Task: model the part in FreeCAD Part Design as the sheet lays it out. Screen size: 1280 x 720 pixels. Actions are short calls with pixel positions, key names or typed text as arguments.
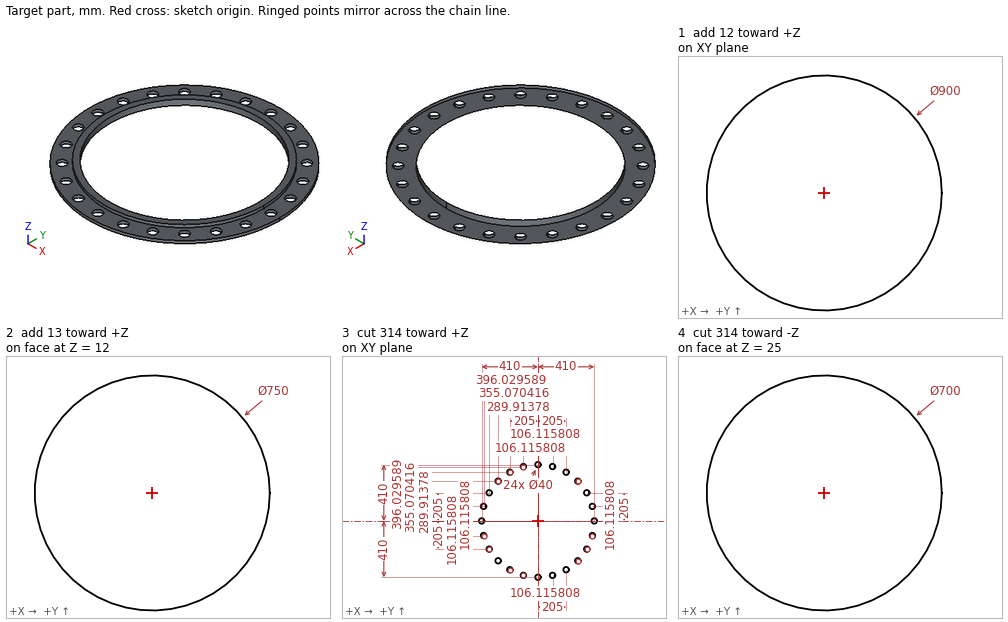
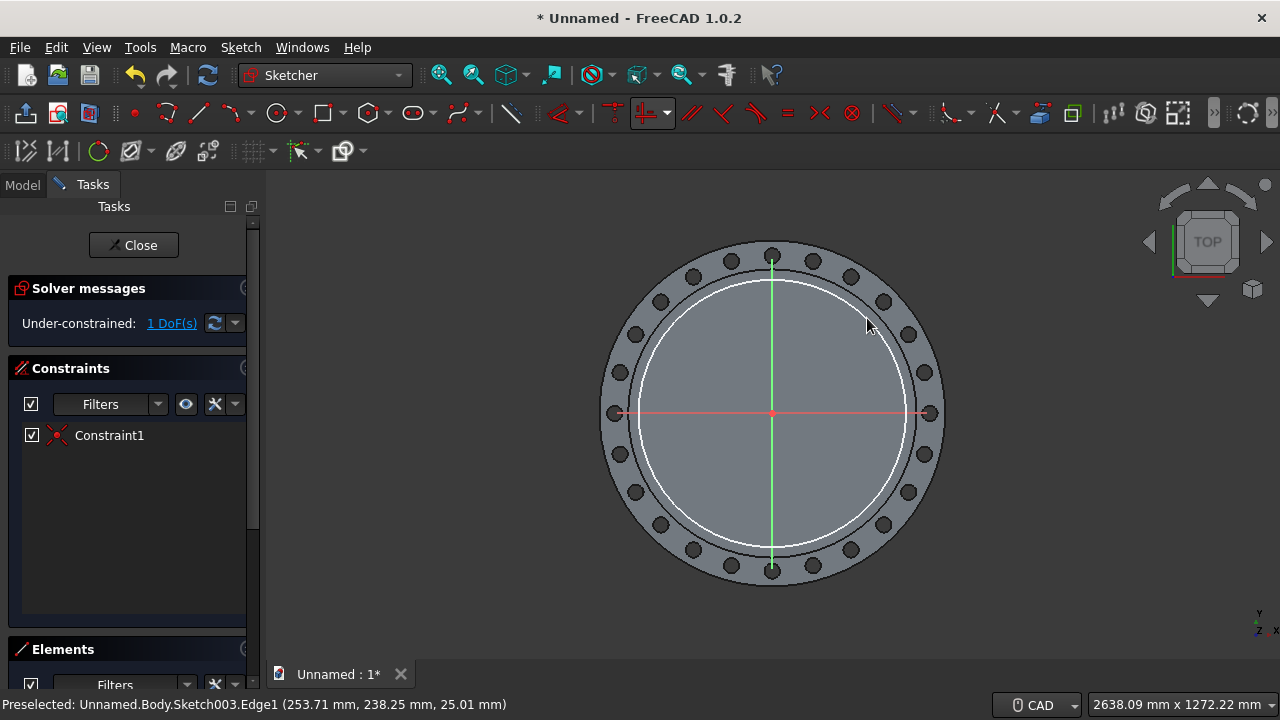
click(558, 114)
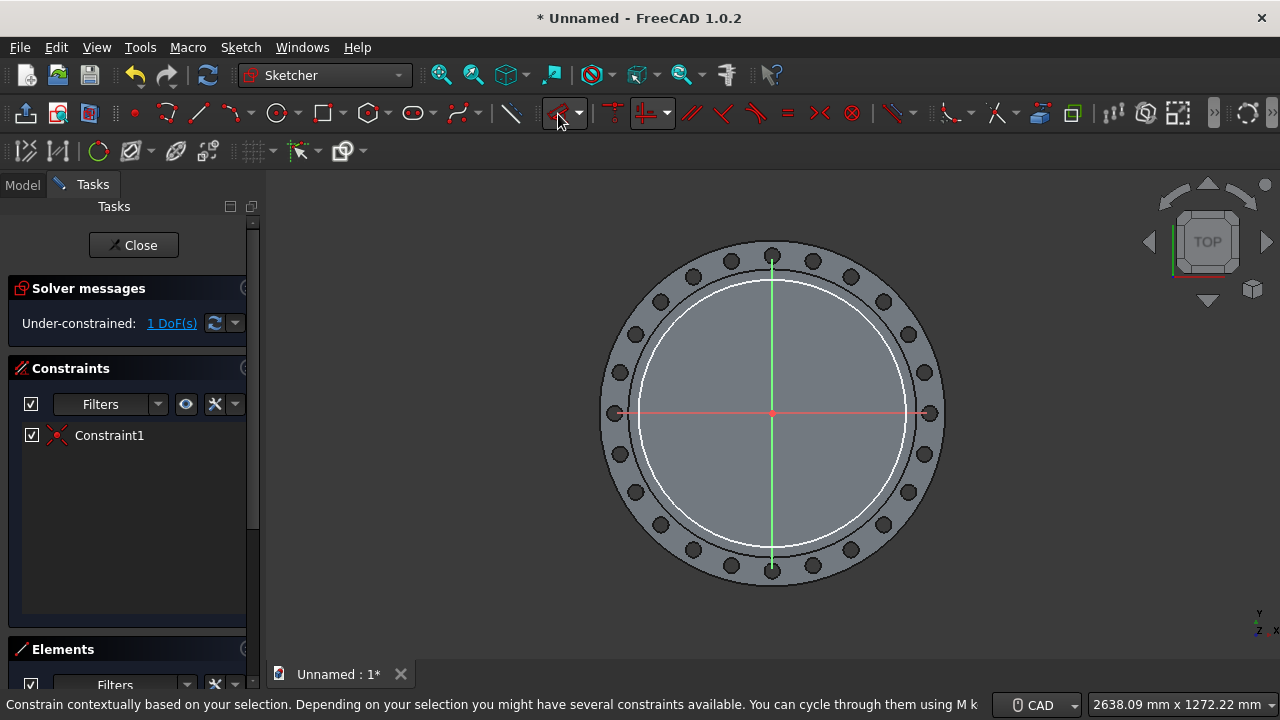
click(867, 319)
click(890, 296)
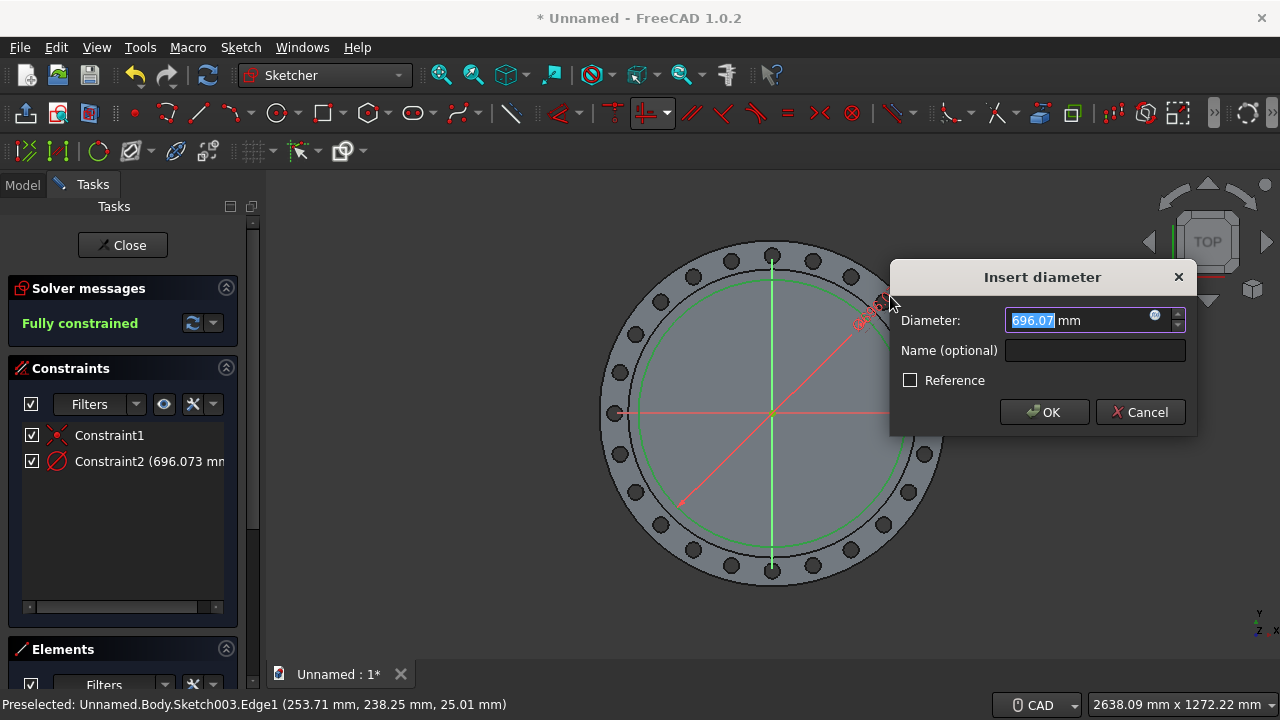
text(700)
key(Return)
key(Escape)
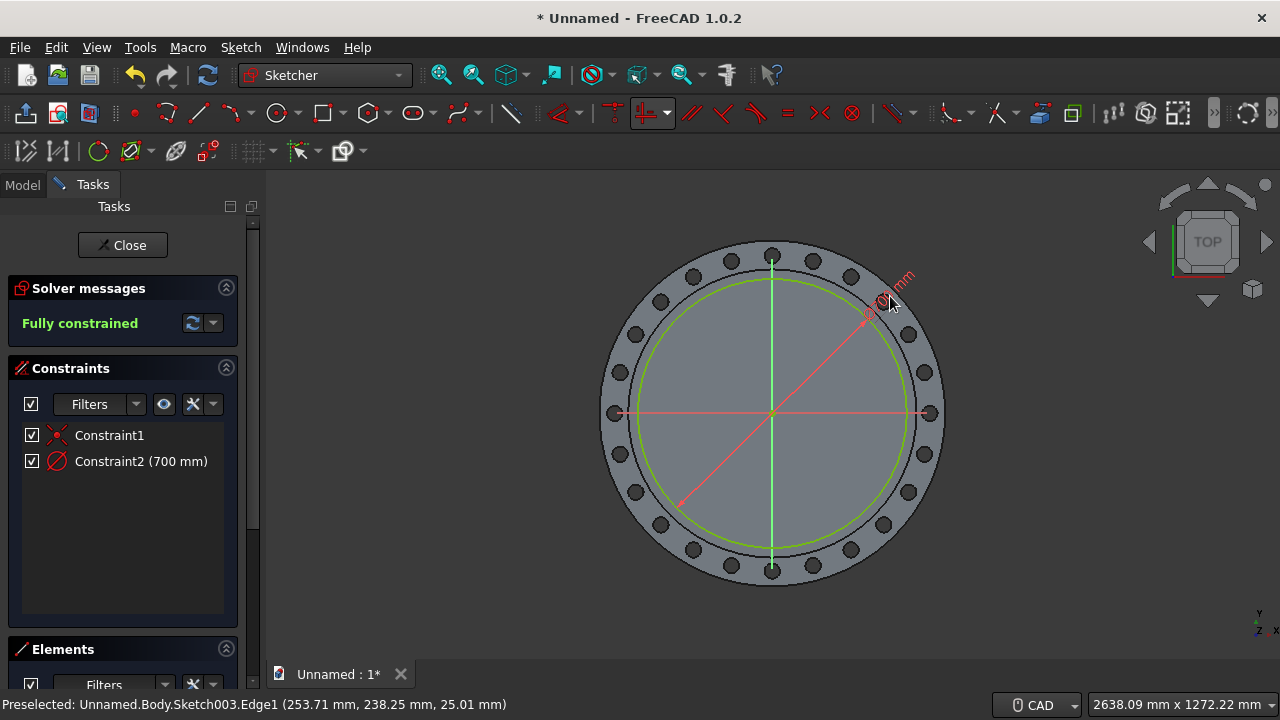
click(123, 245)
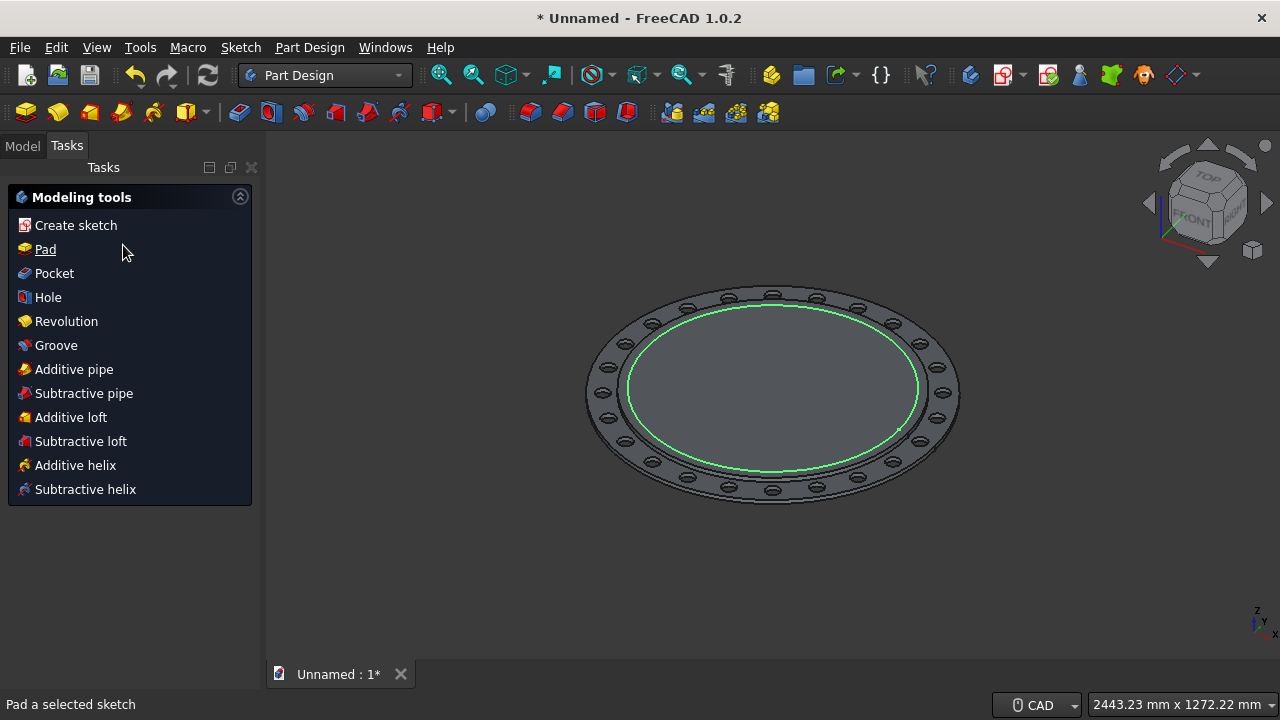
click(240, 112)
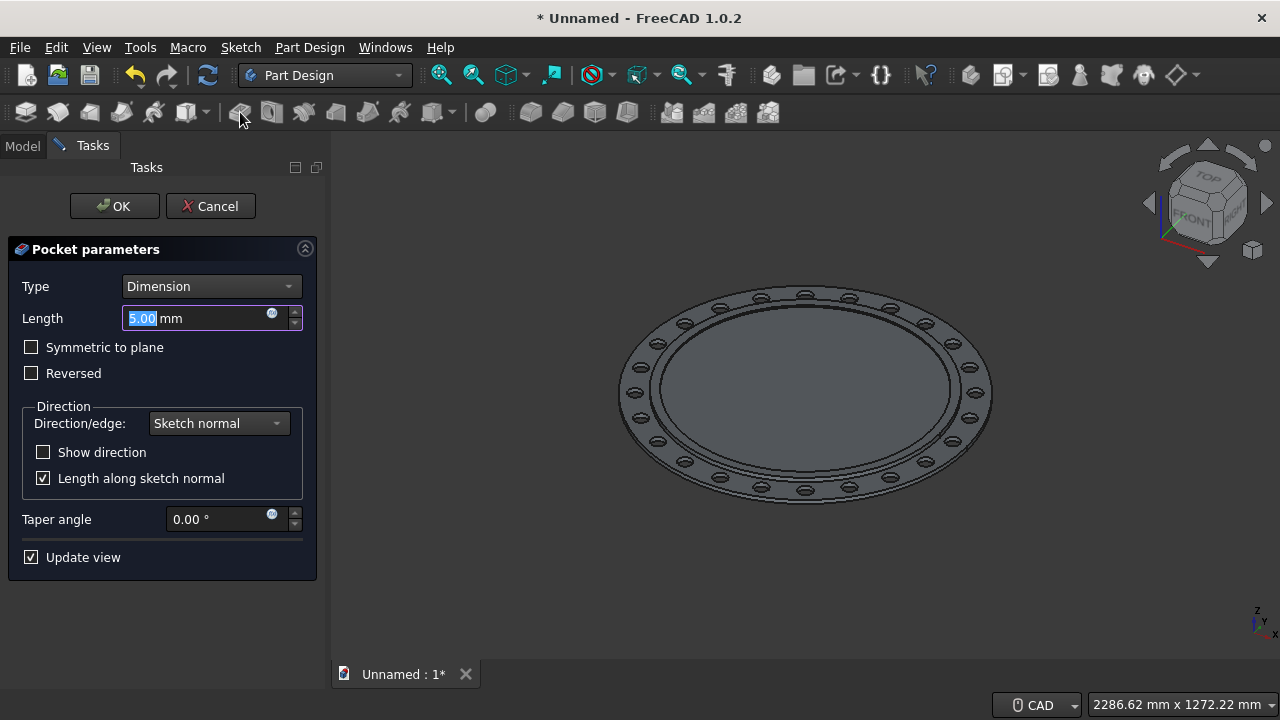
text(314)
key(Tab)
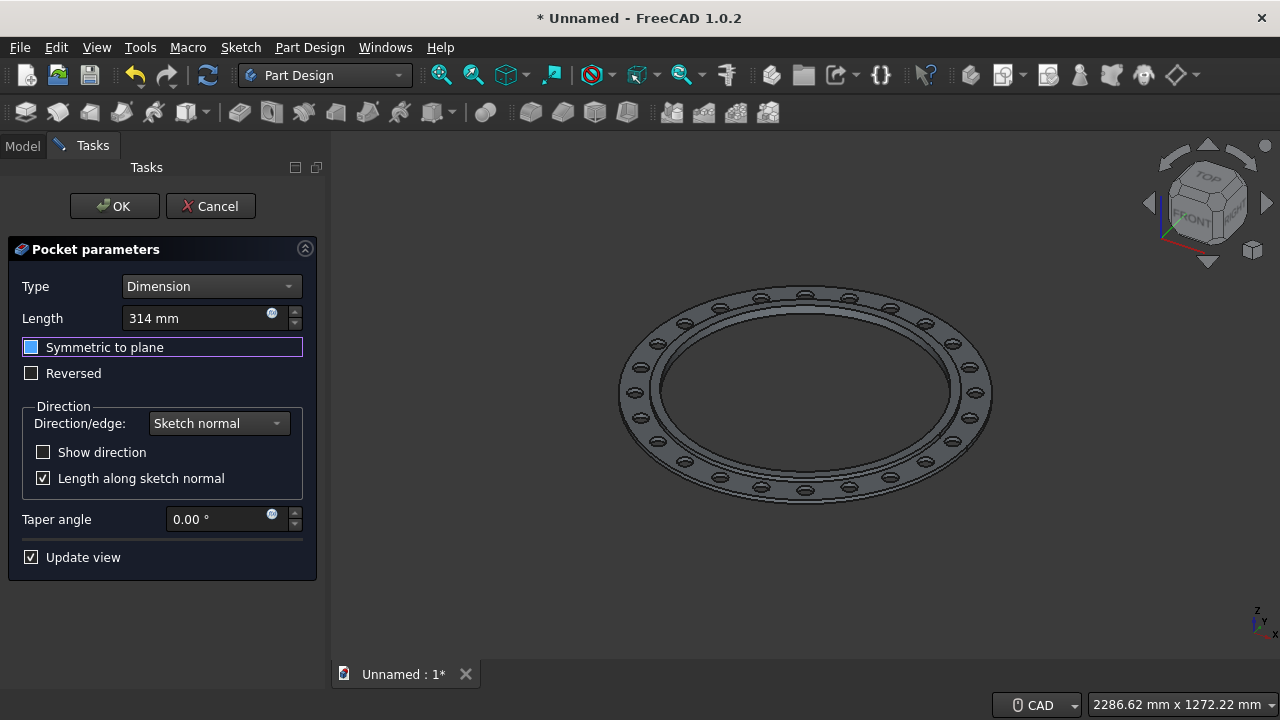
click(115, 206)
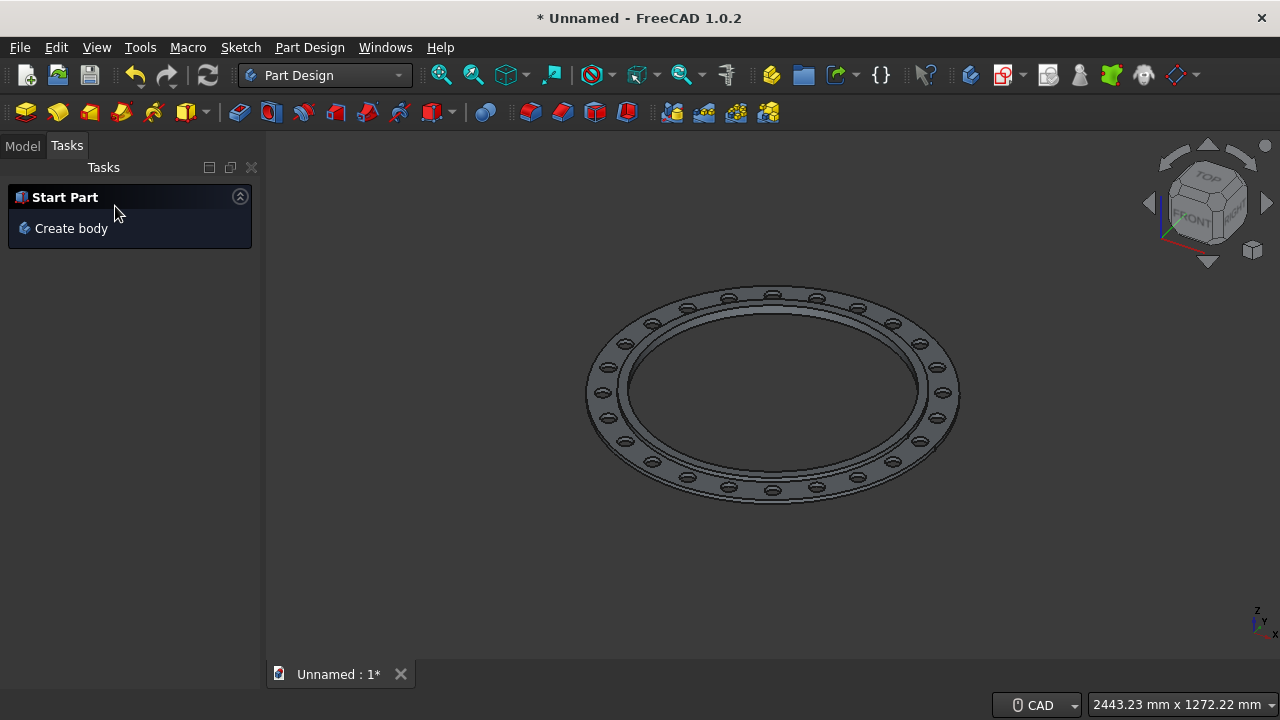
key(0)